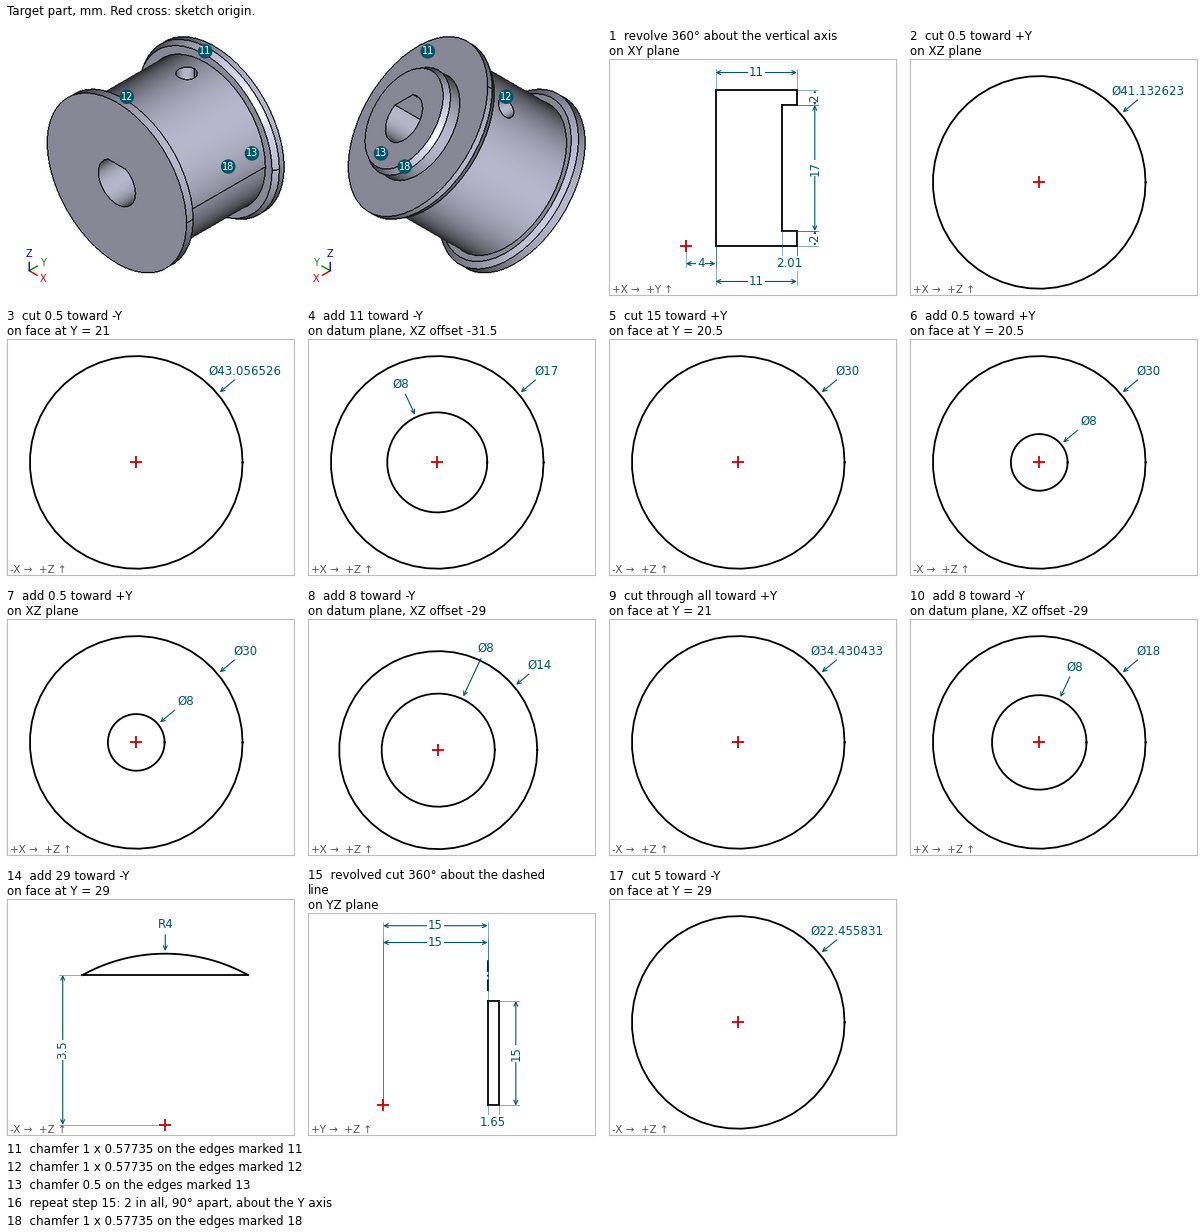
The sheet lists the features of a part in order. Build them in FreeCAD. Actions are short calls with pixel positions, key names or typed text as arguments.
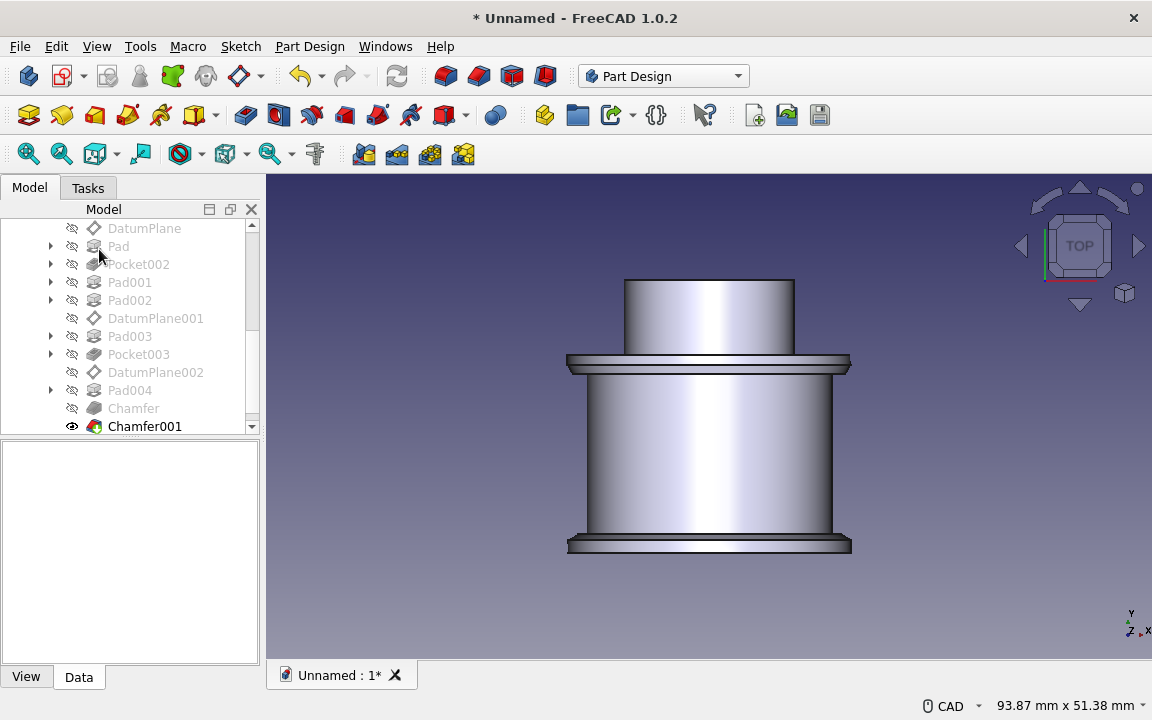
click(640, 279)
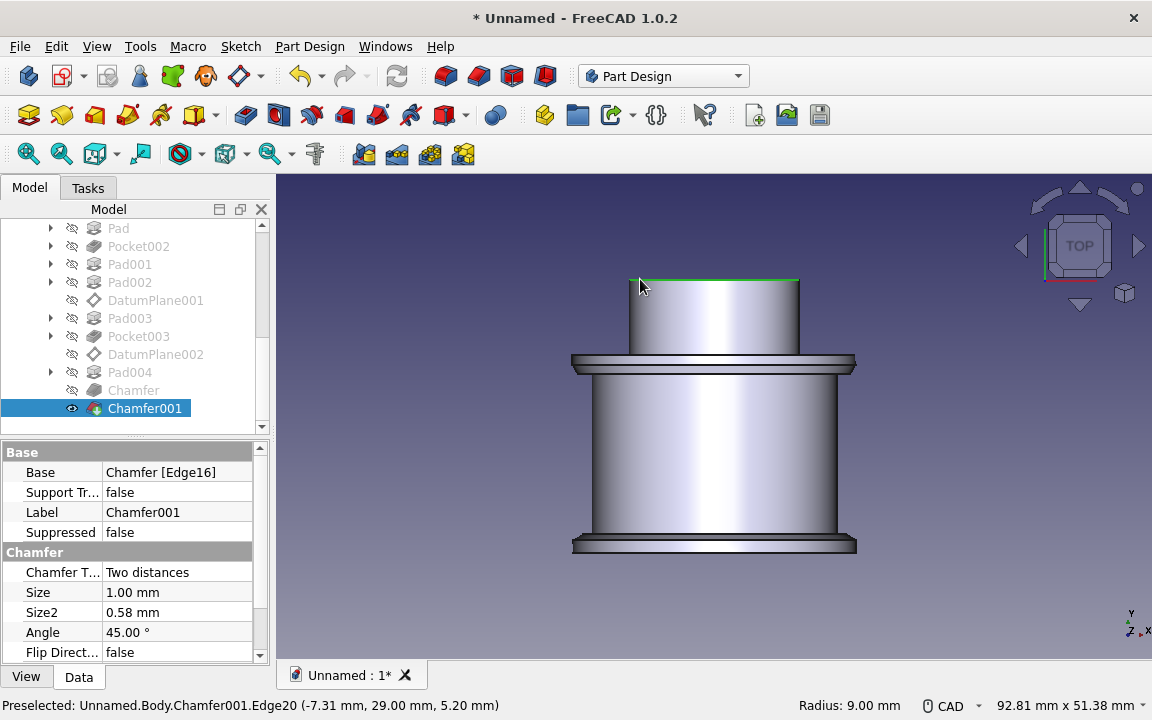
click(479, 76)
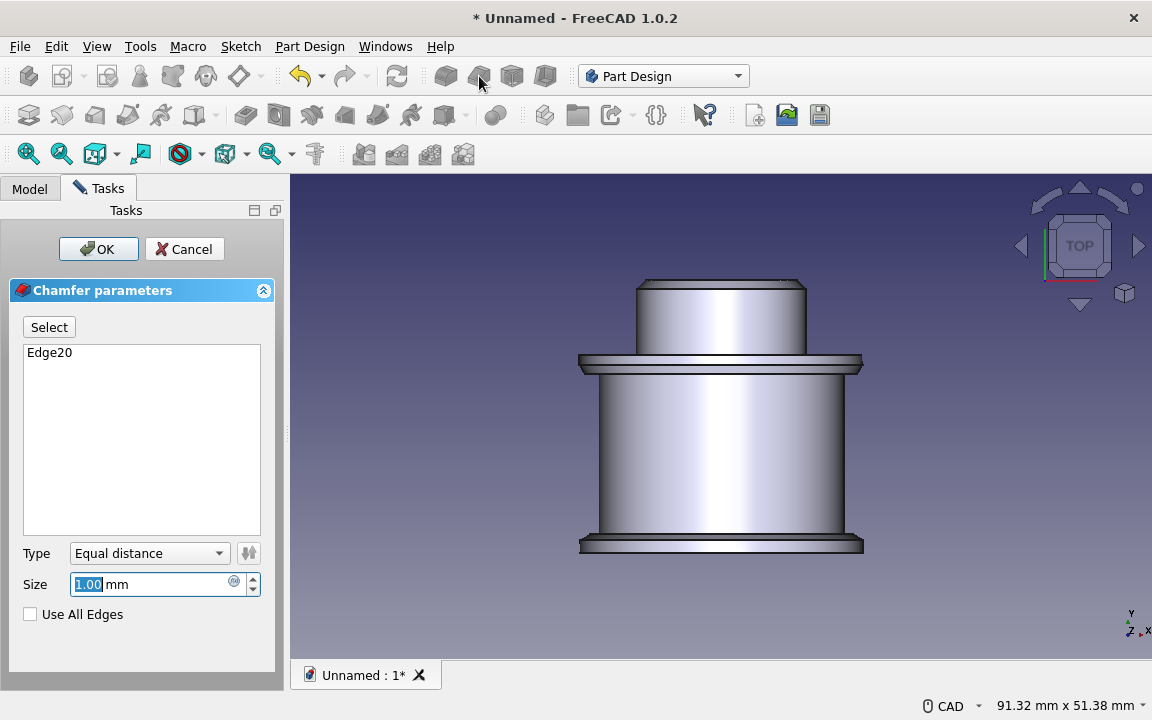
text(0.5)
key(Tab)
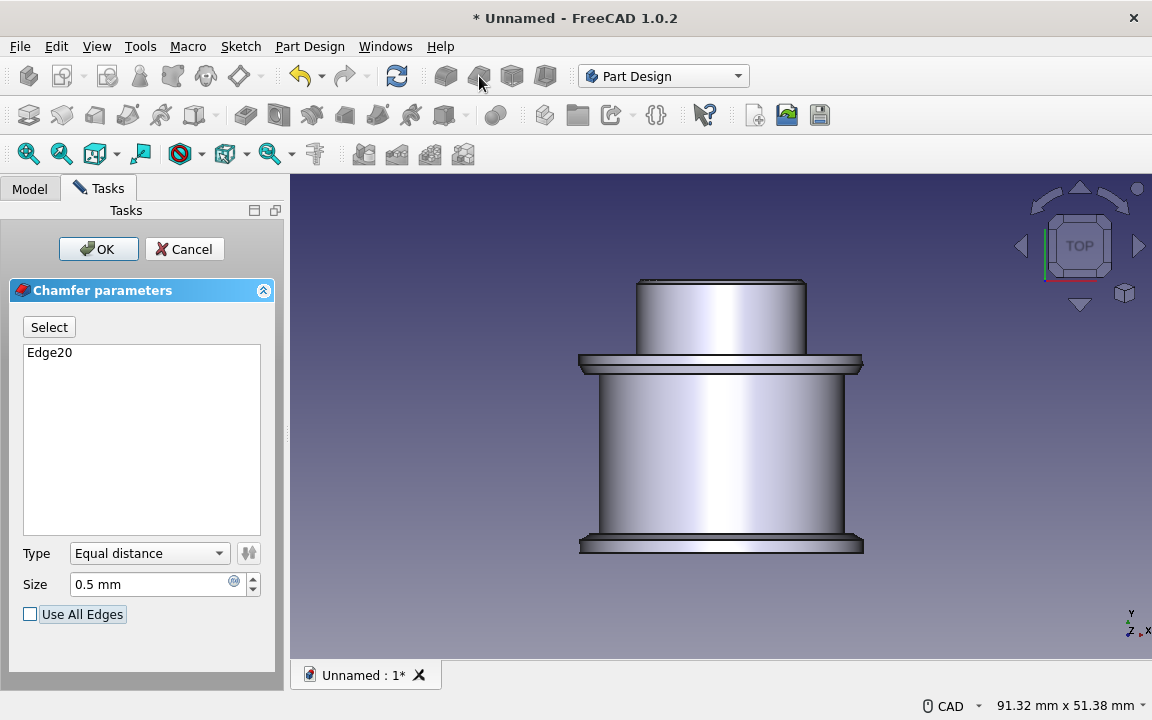
click(99, 249)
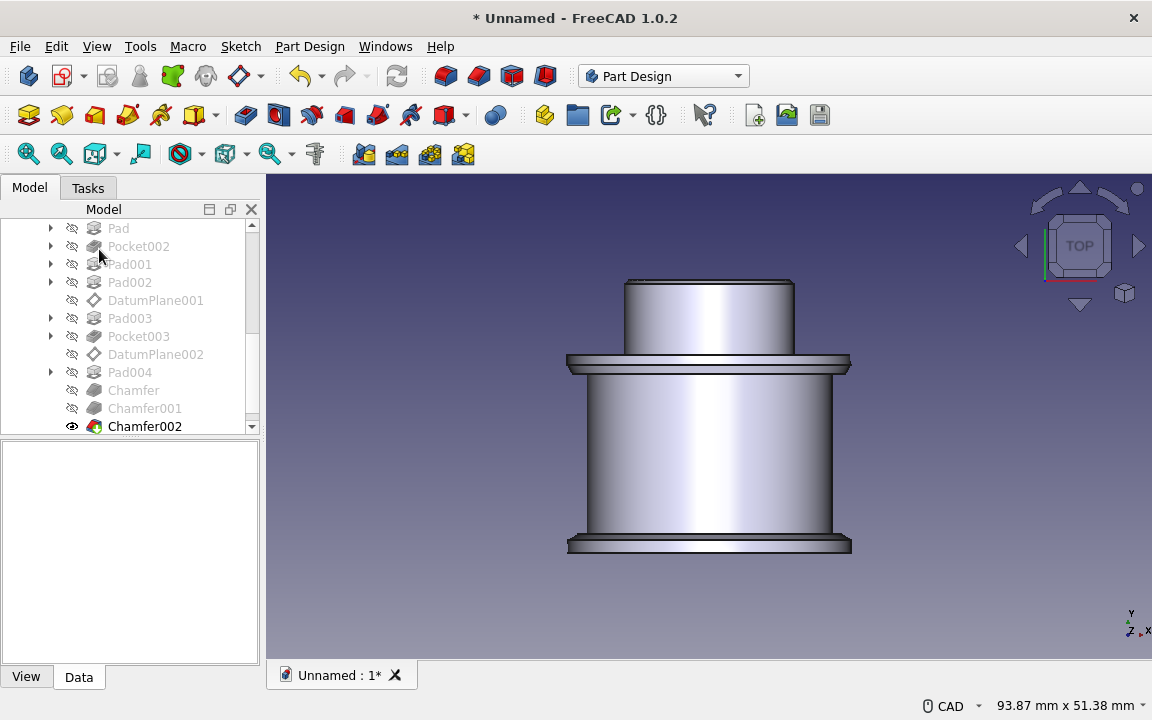
key(4)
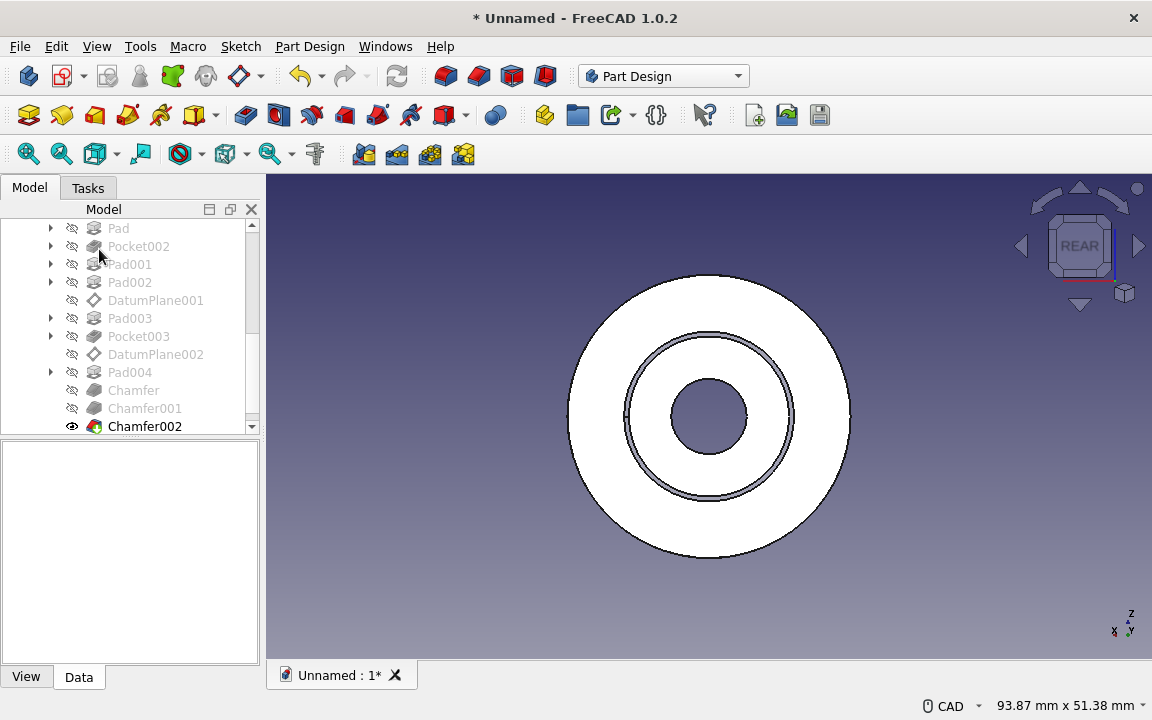
click(755, 461)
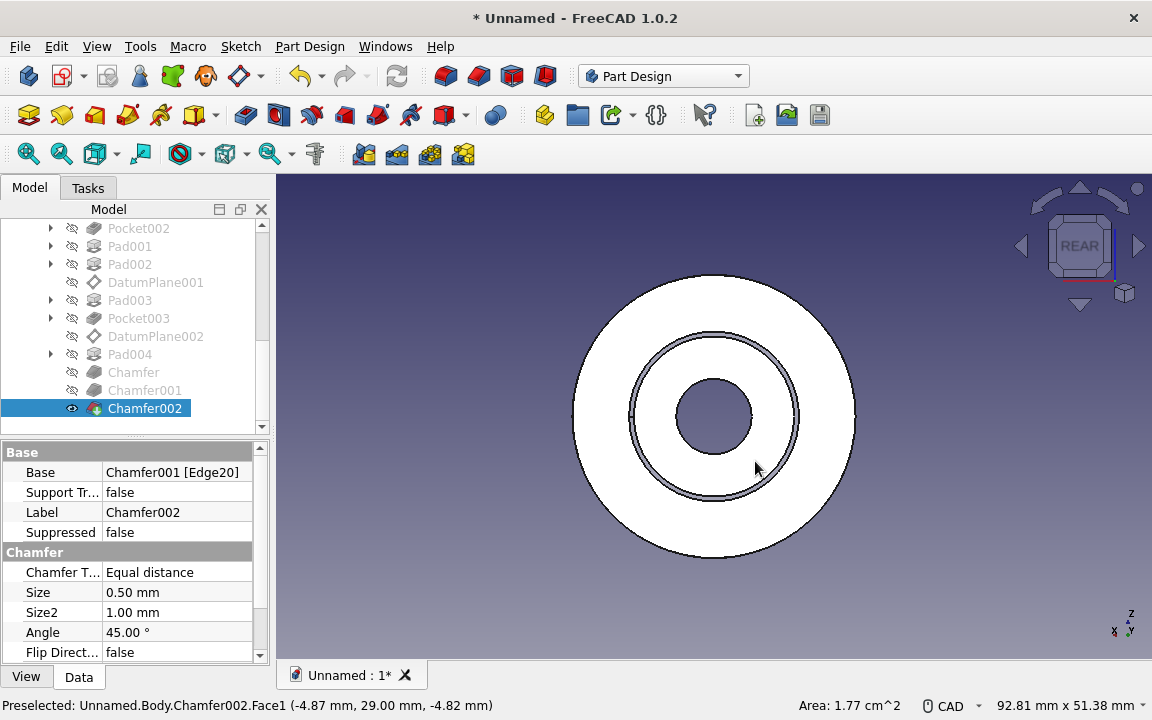
click(62, 76)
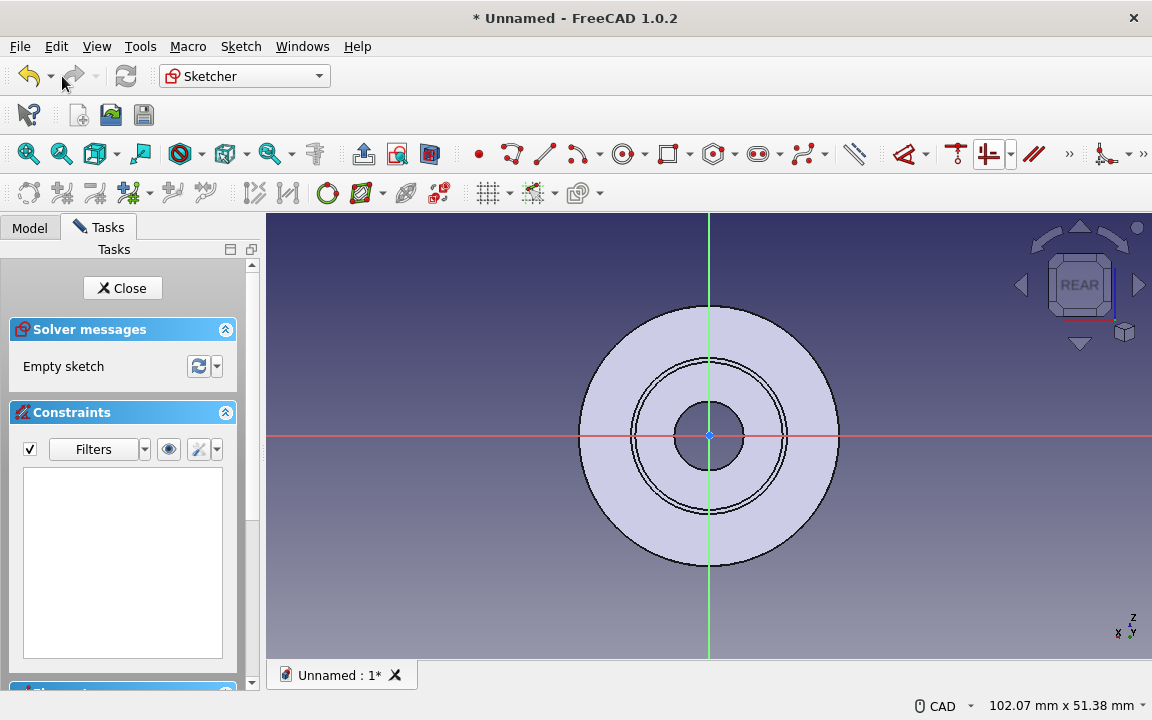
scroll(720, 416, up, 10)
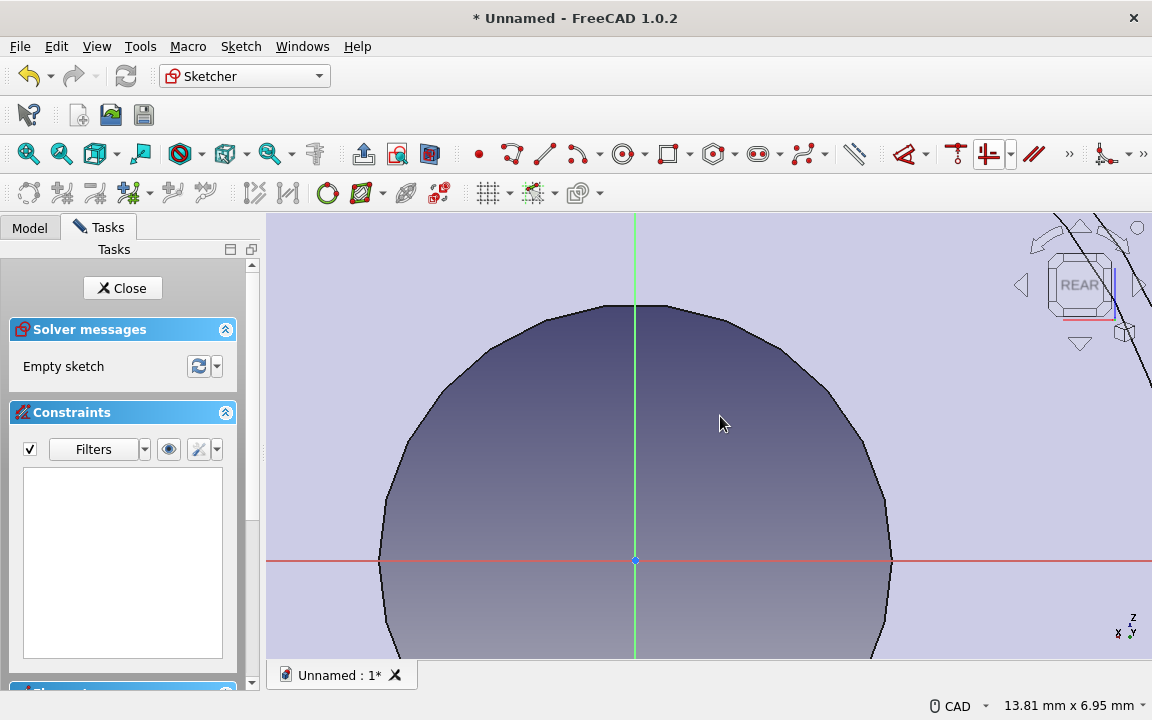
click(545, 154)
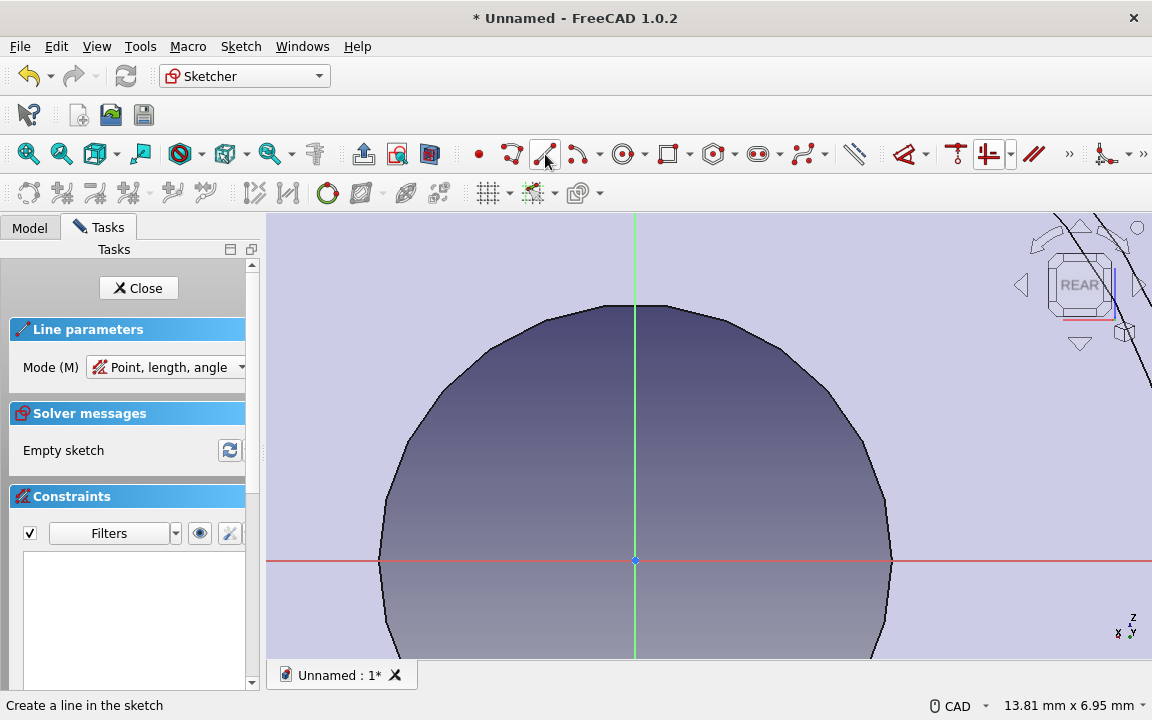
click(511, 336)
click(760, 336)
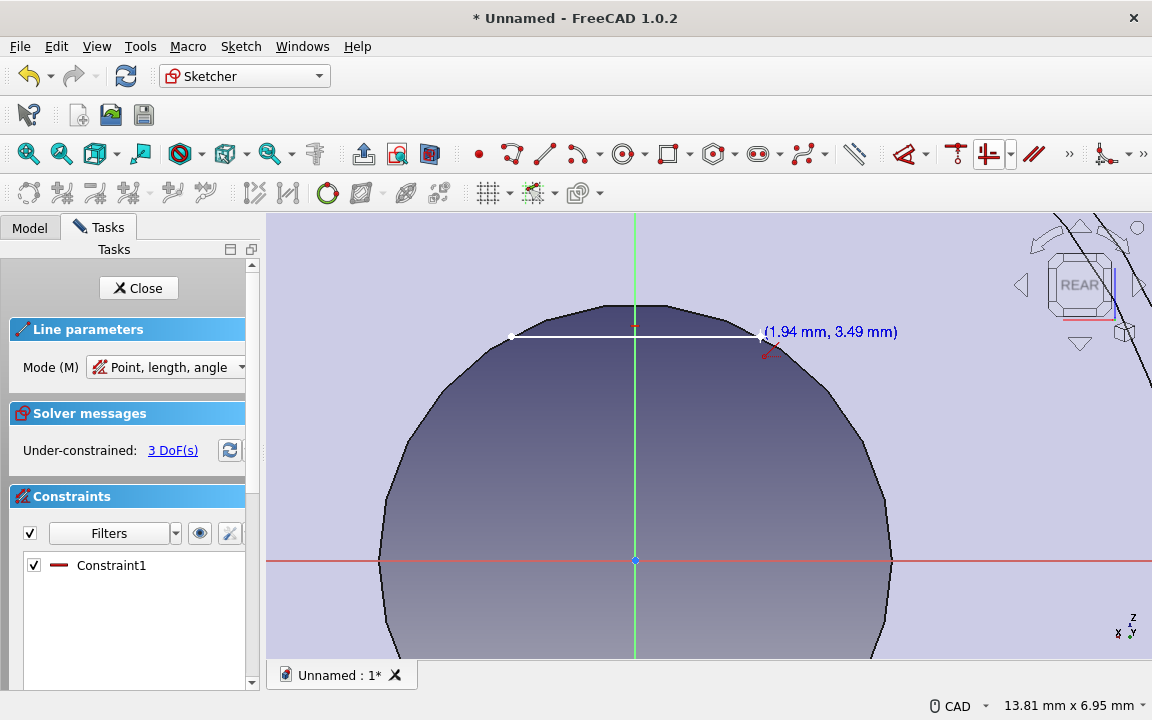
key(g)
key(3)
key(a)